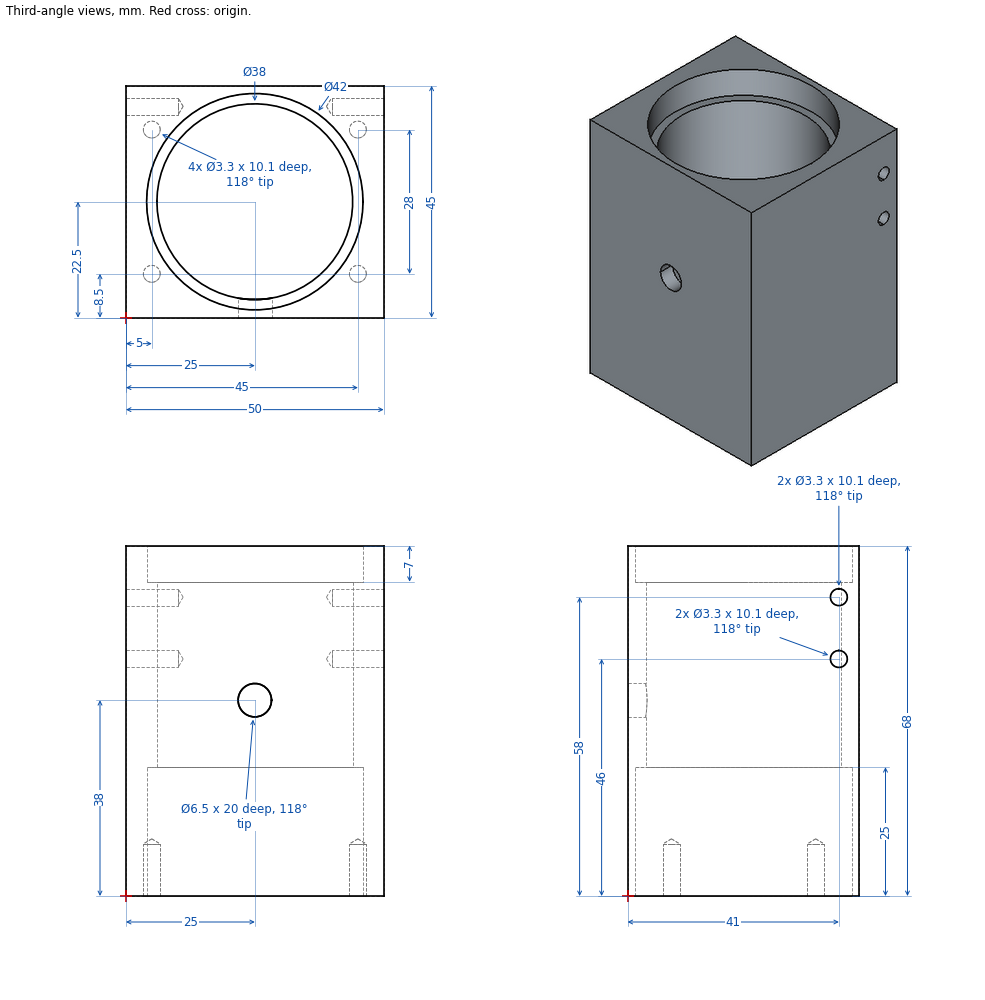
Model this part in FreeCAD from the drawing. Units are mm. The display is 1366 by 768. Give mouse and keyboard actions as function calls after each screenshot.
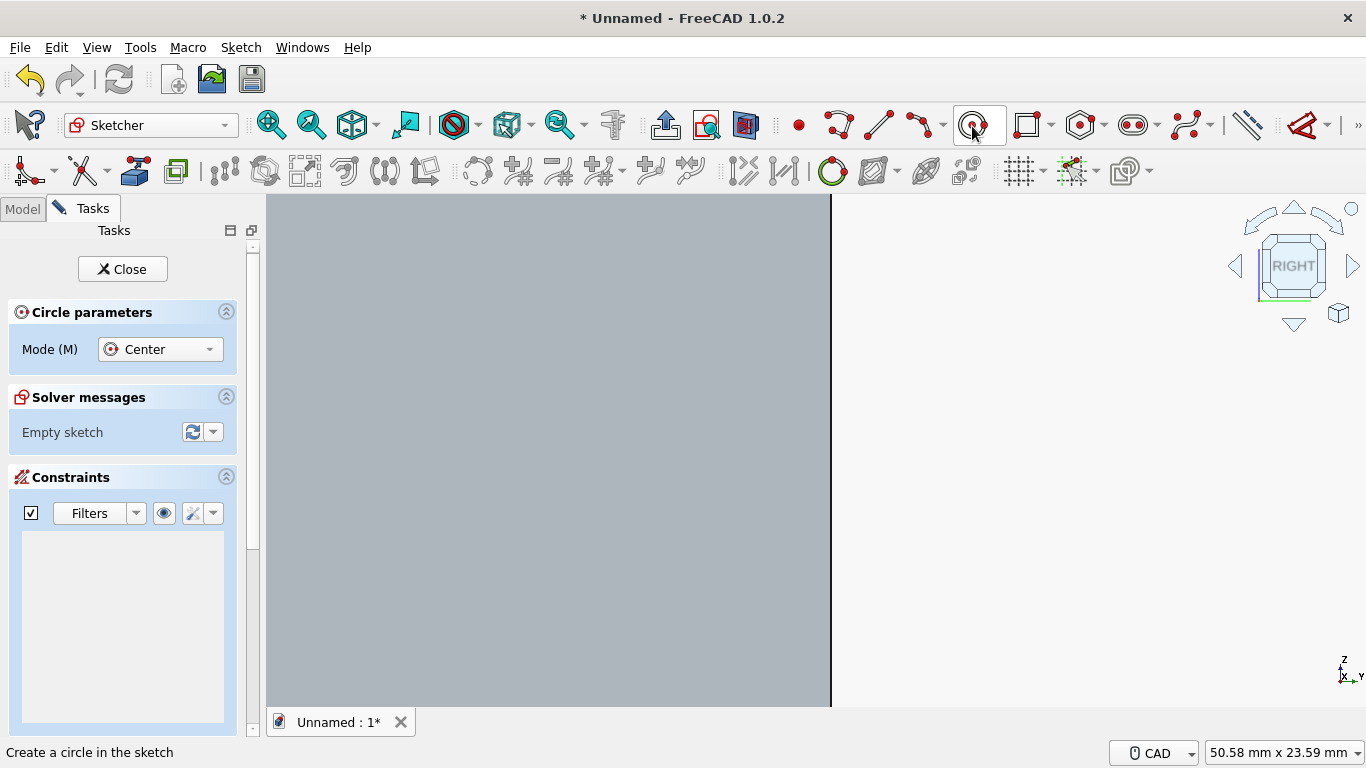
click(744, 320)
move(770, 295)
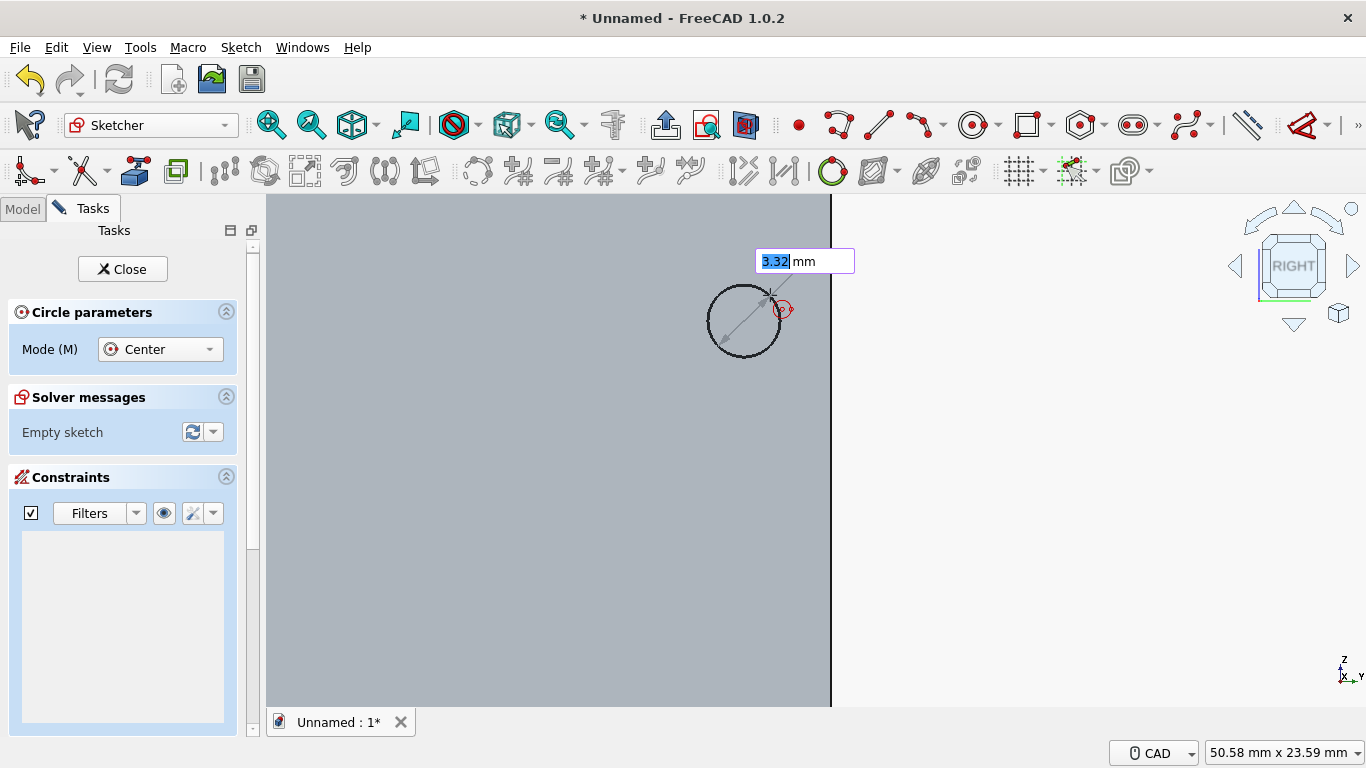
text(3.3)
key(Return)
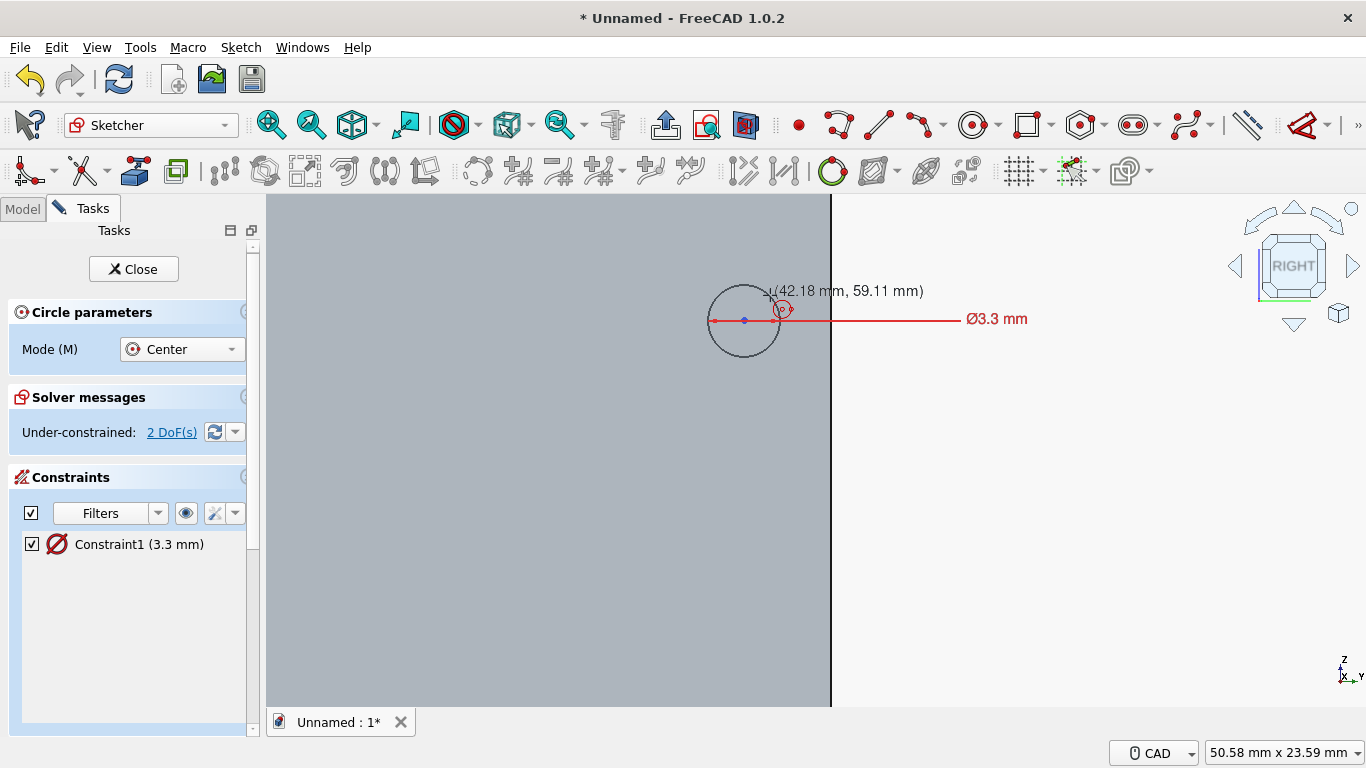
click(744, 581)
move(770, 556)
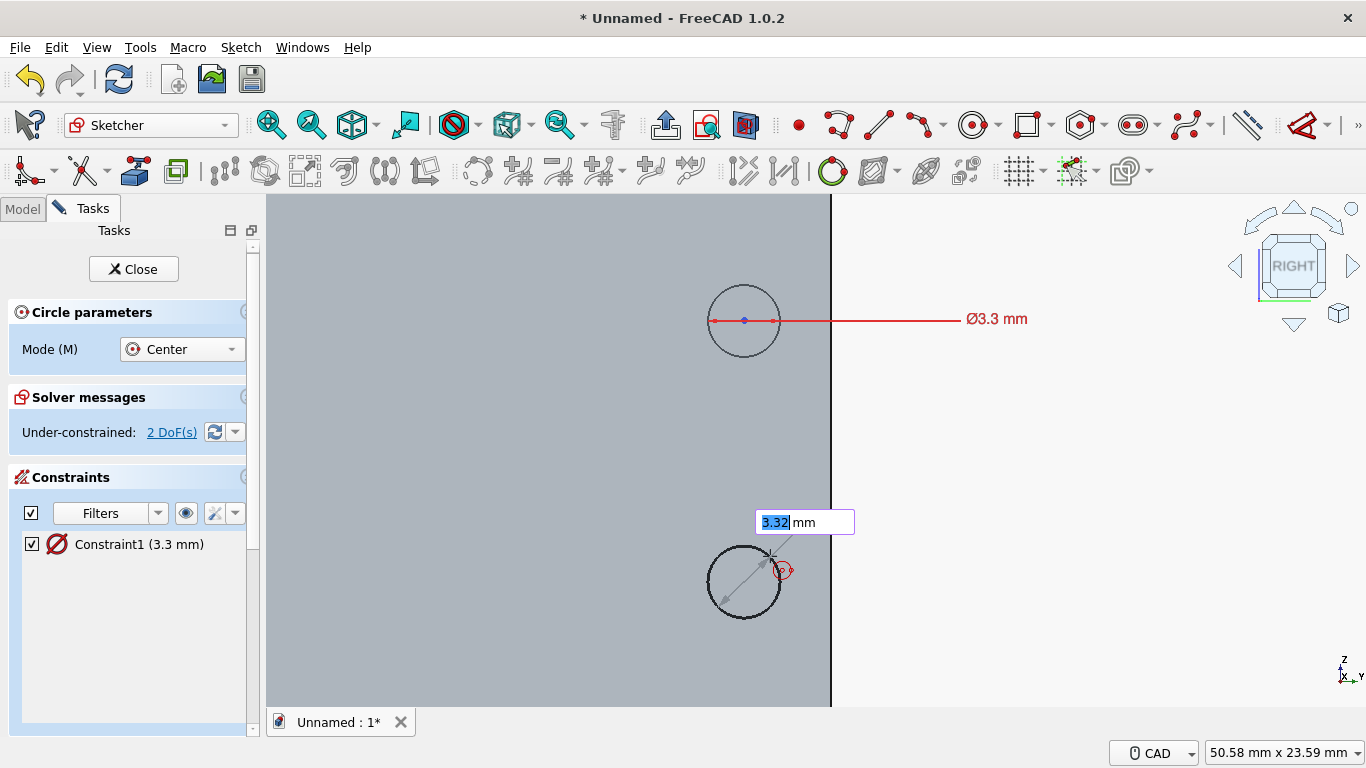
text(3.3)
key(Return)
key(Escape)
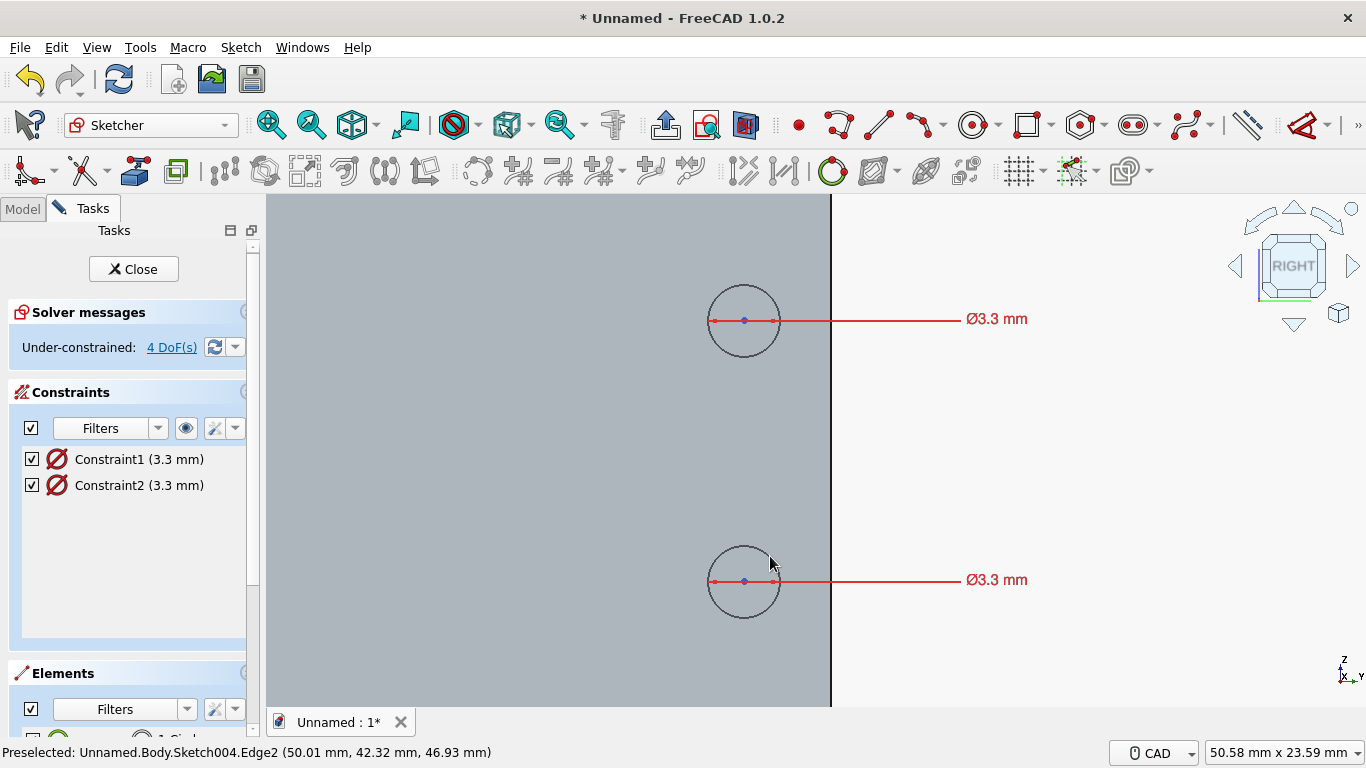
click(744, 321)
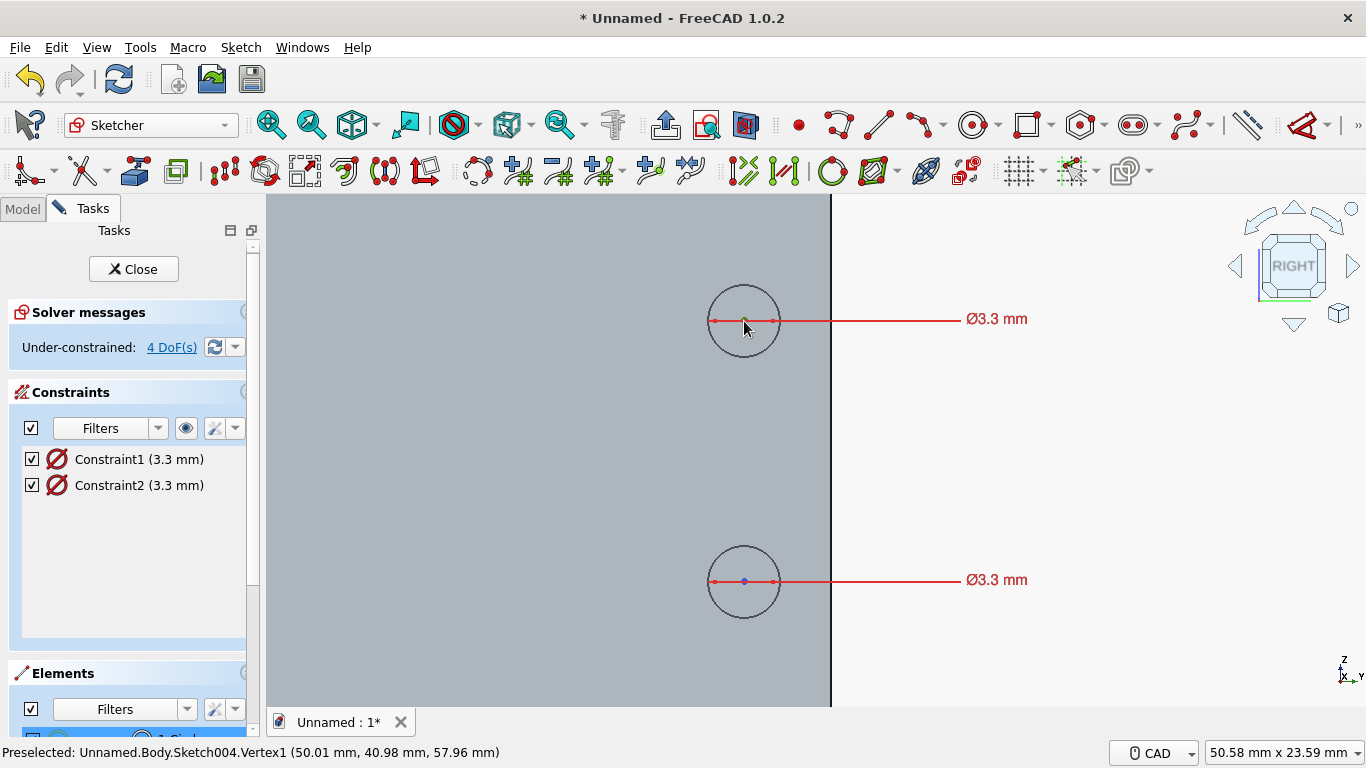
click(744, 582)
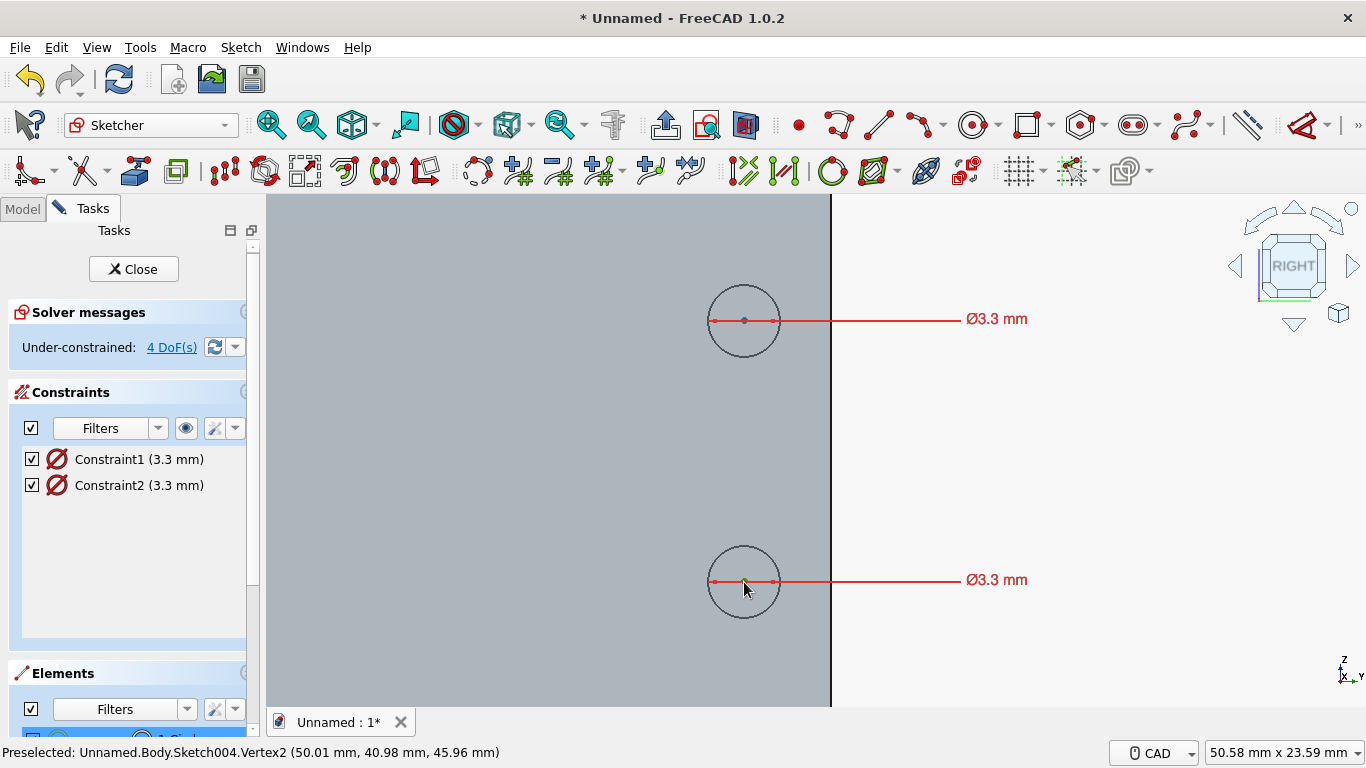
key(v)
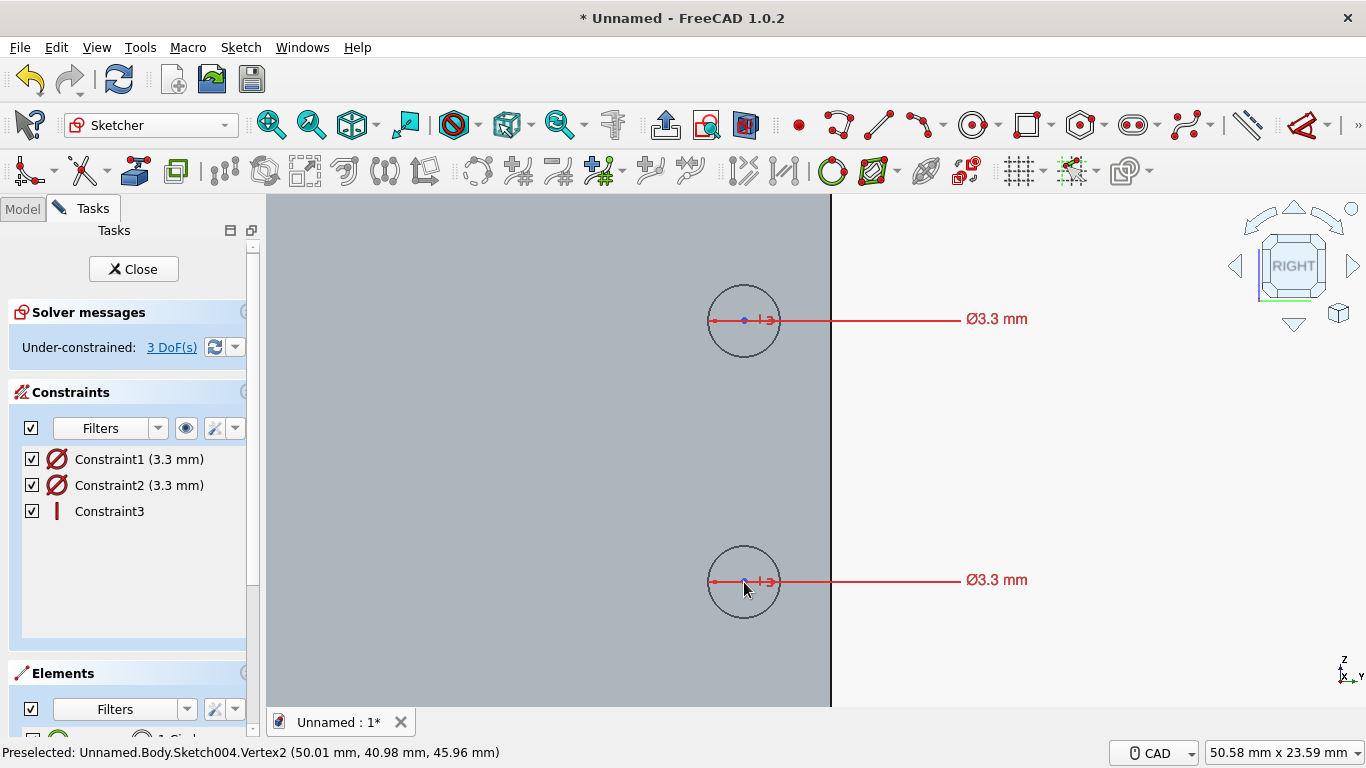
key(d)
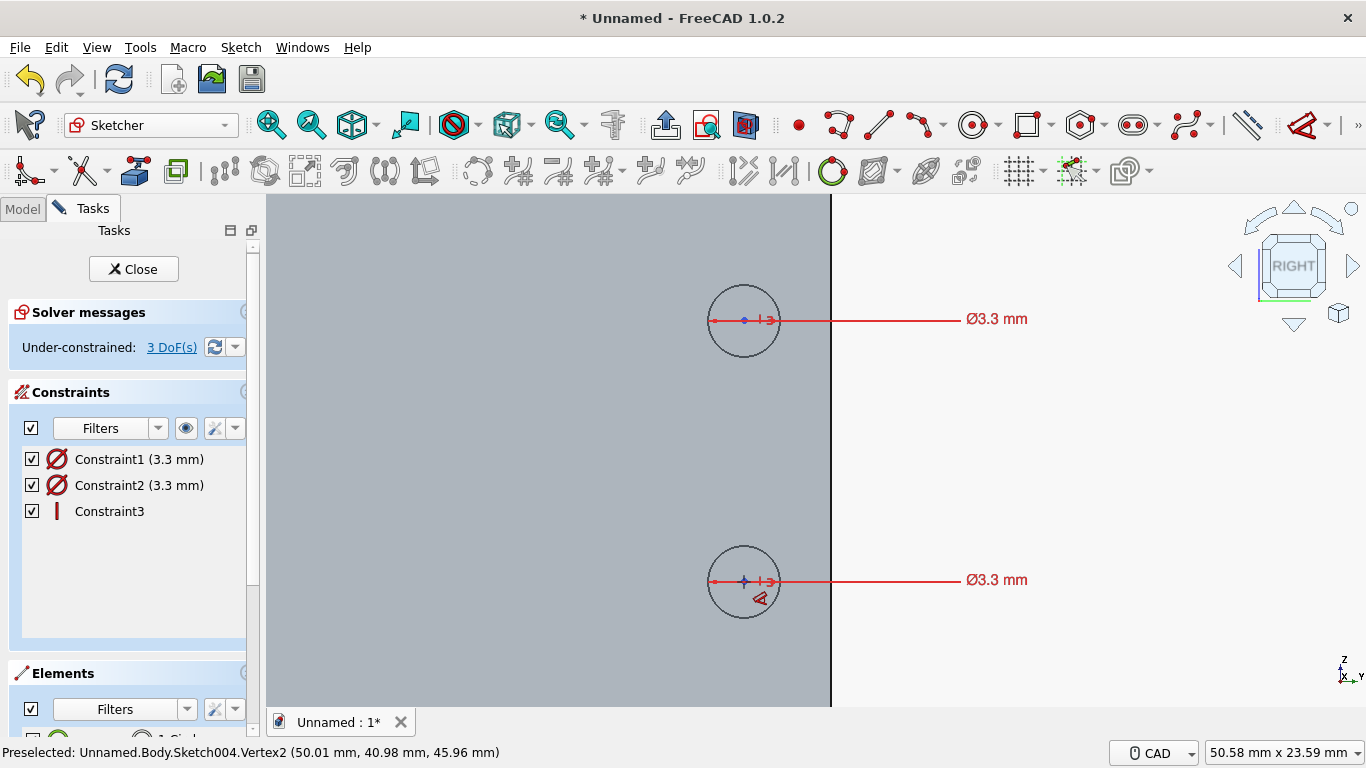
click(744, 321)
click(519, 287)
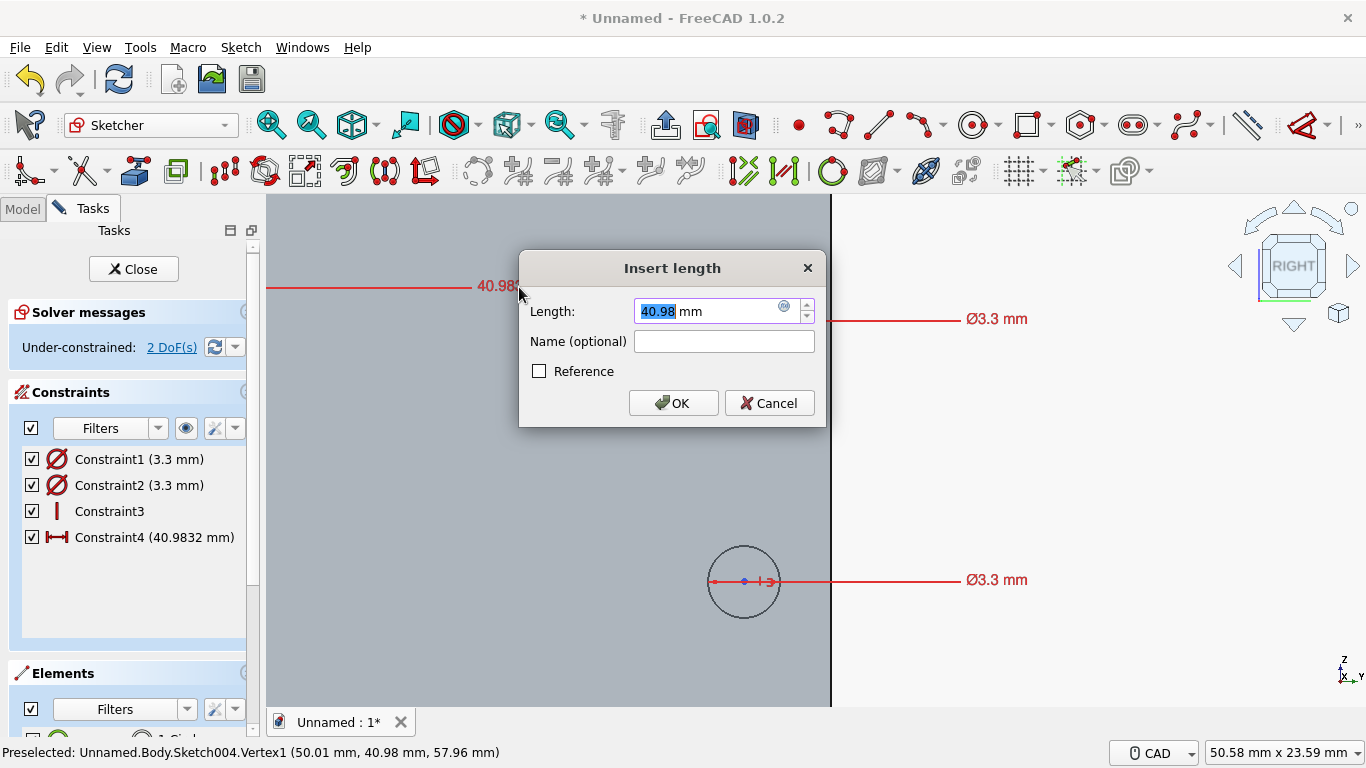
text(41)
key(Return)